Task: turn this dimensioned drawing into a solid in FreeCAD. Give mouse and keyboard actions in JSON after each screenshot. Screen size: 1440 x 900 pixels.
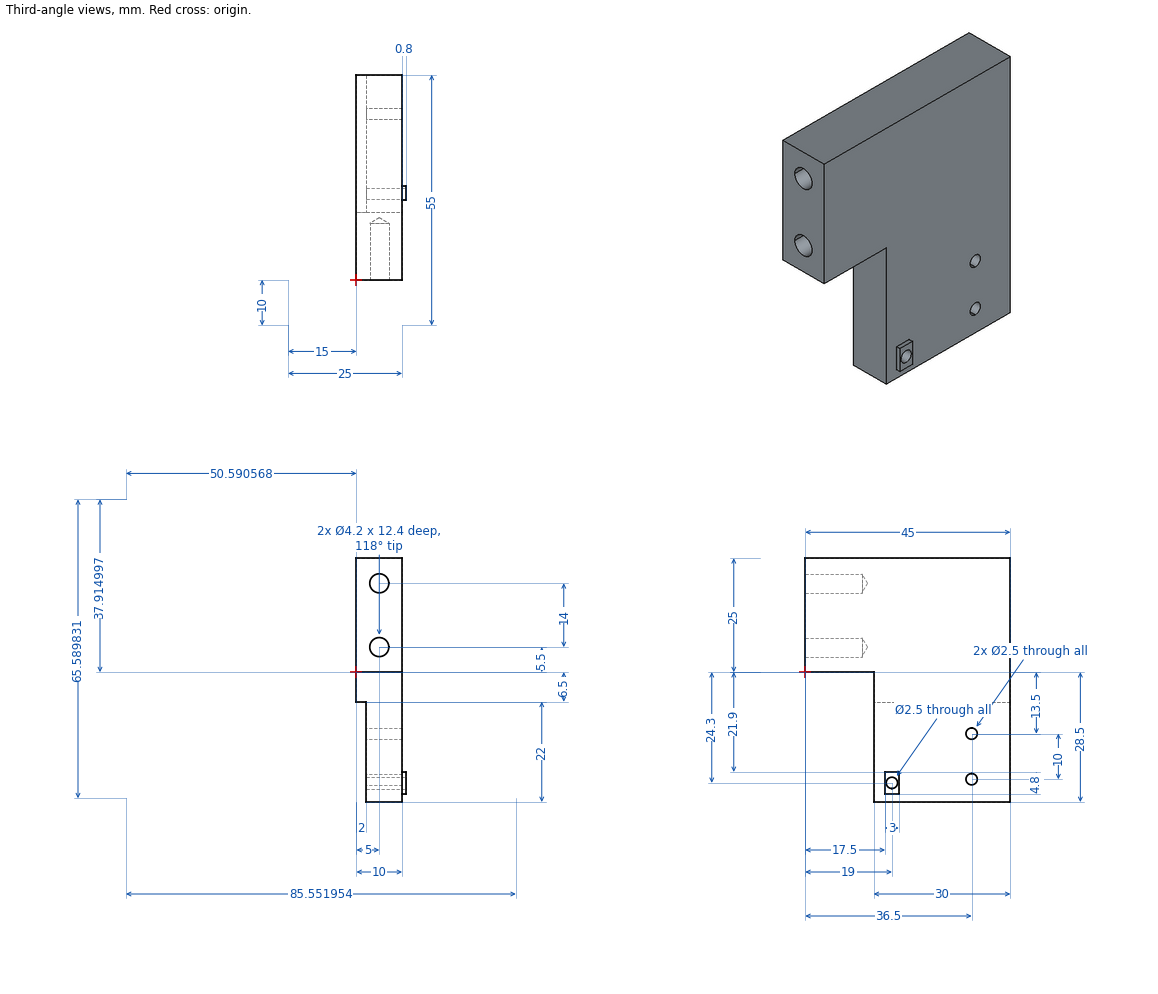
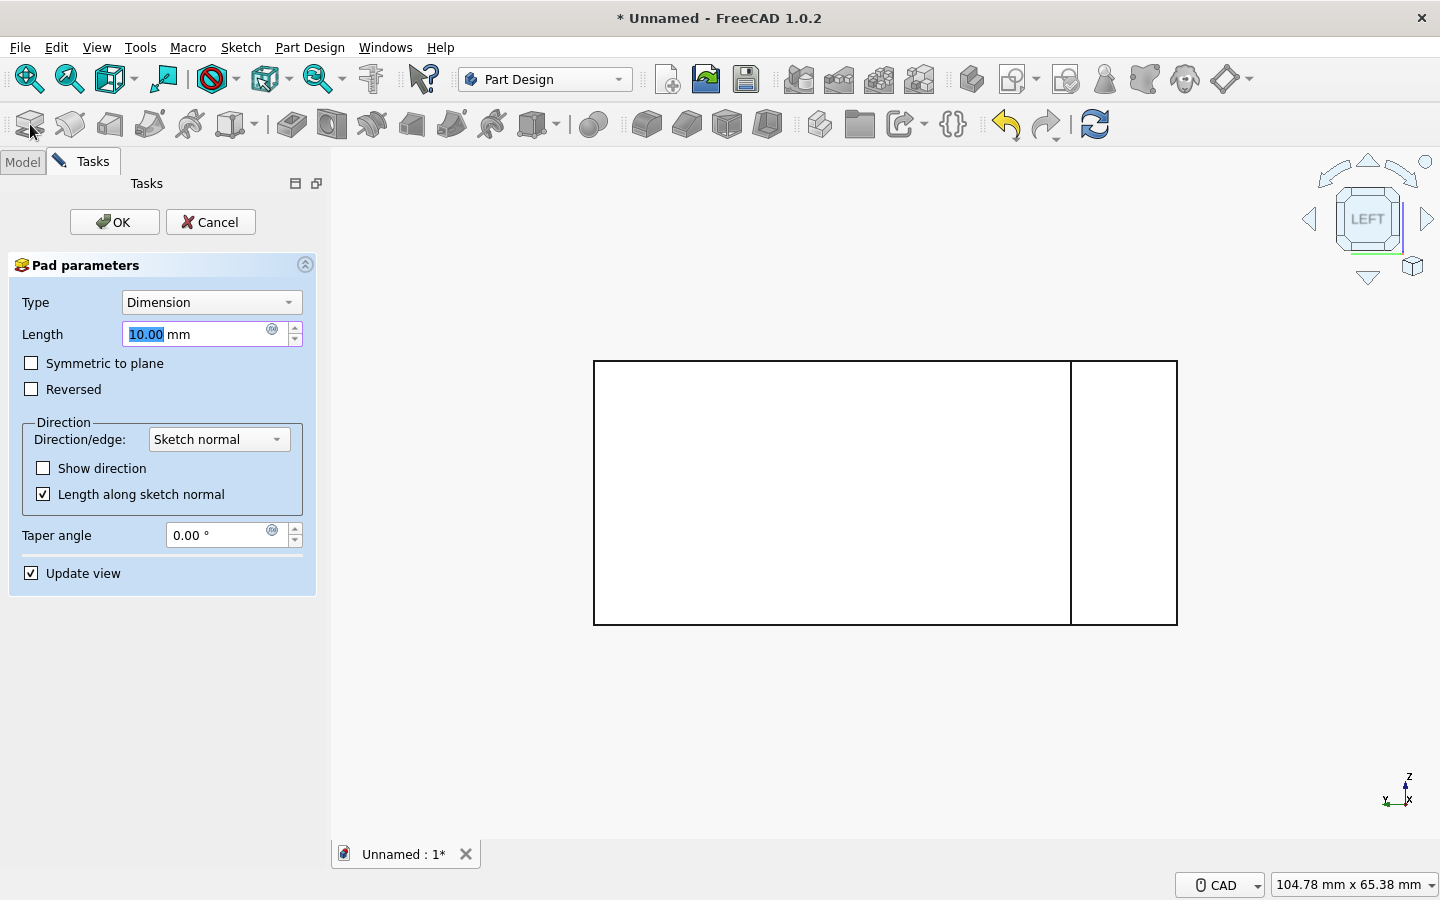
{"action": "type", "text": "10"}
{"action": "key", "text": "Tab"}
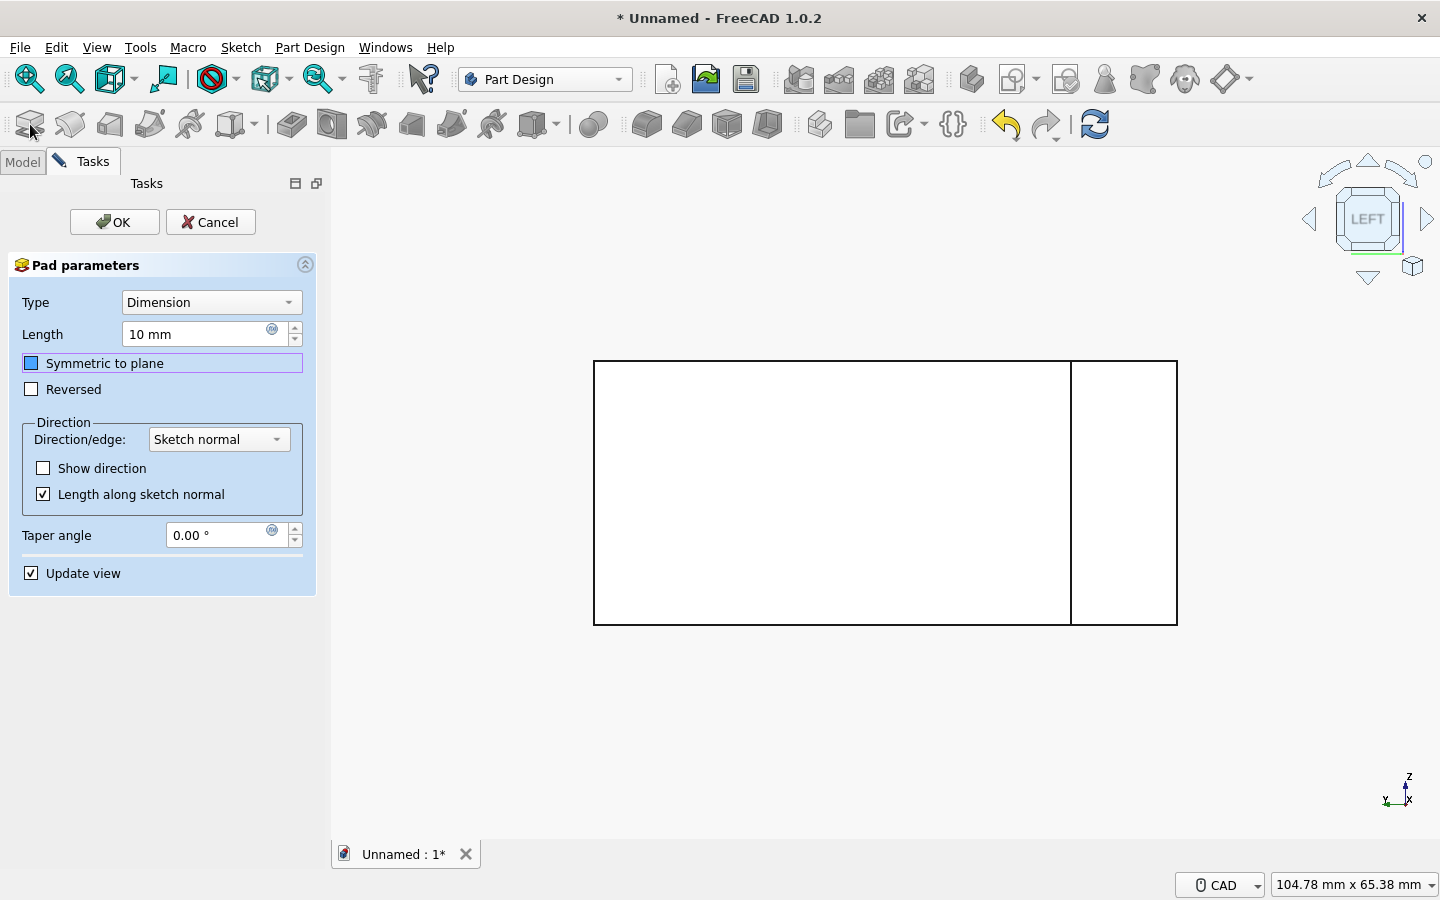
{"action": "left_click", "coordinate": [30, 389]}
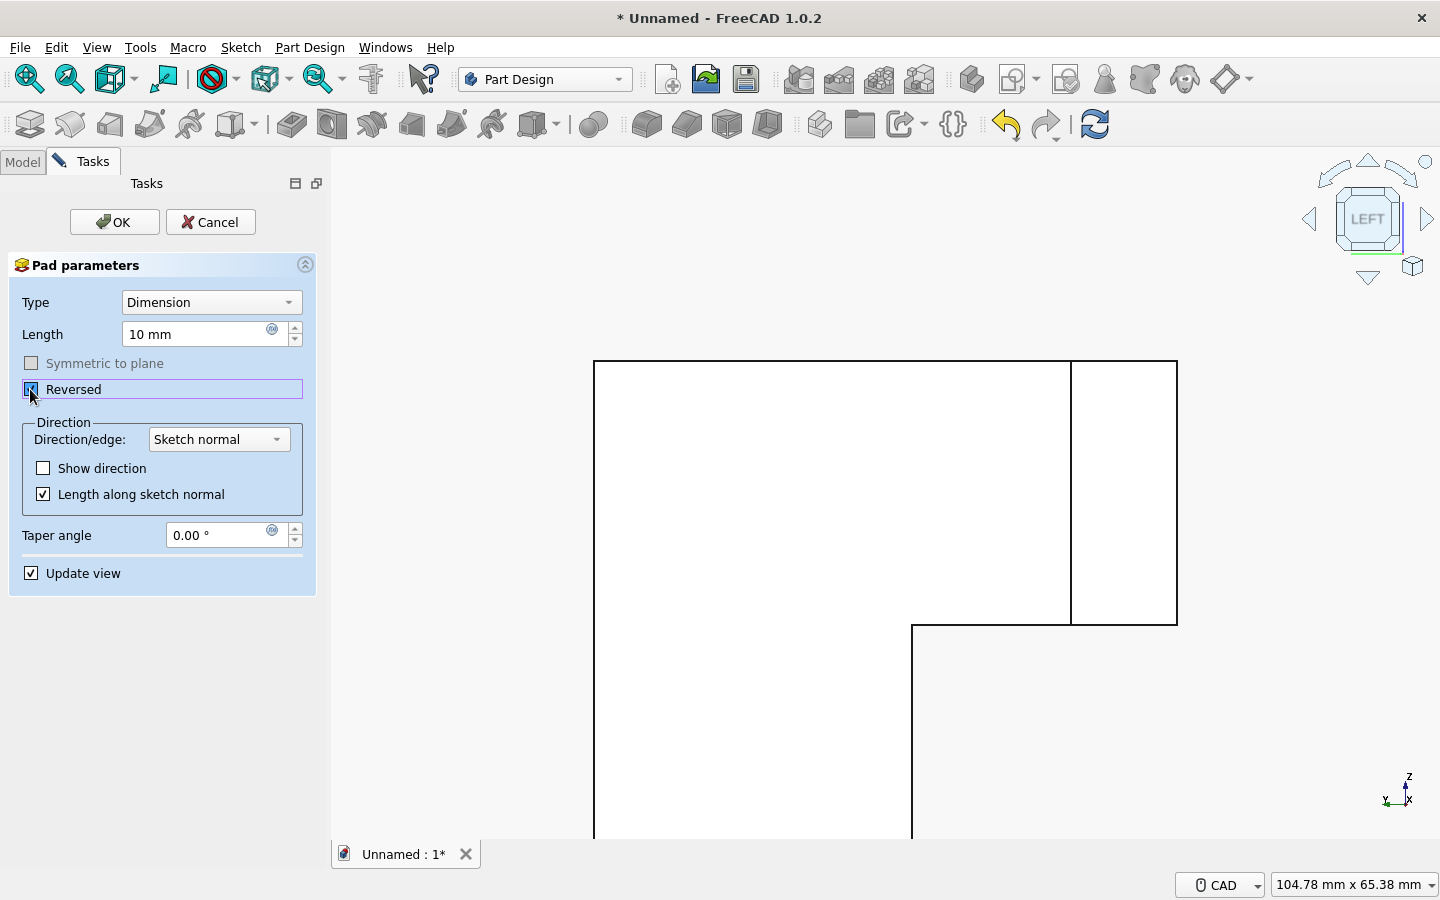
{"action": "left_click", "coordinate": [115, 222]}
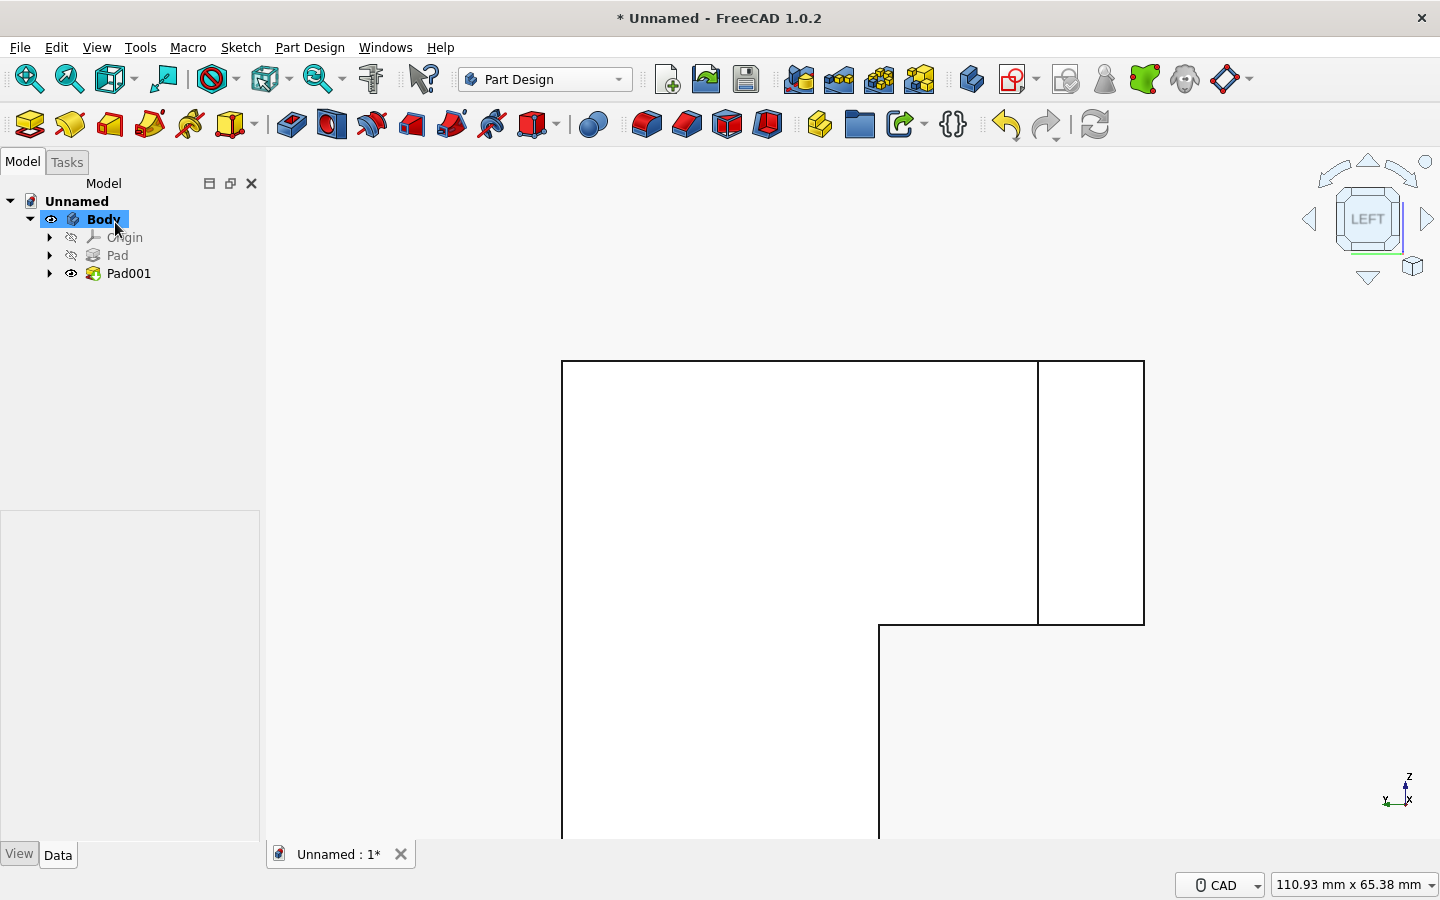
{"action": "key", "text": "v f"}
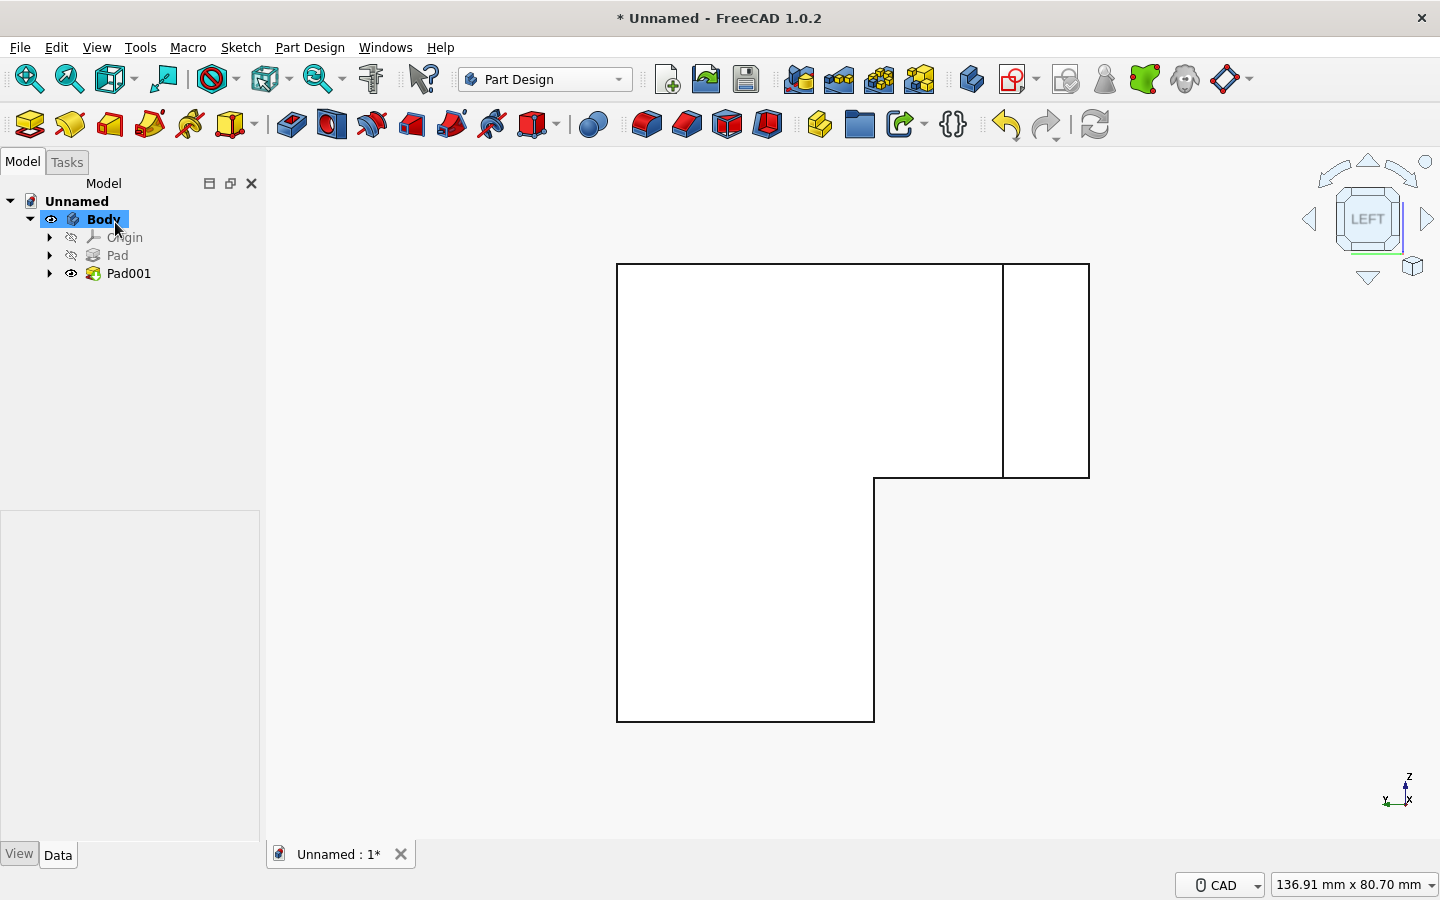
{"action": "key", "text": "4"}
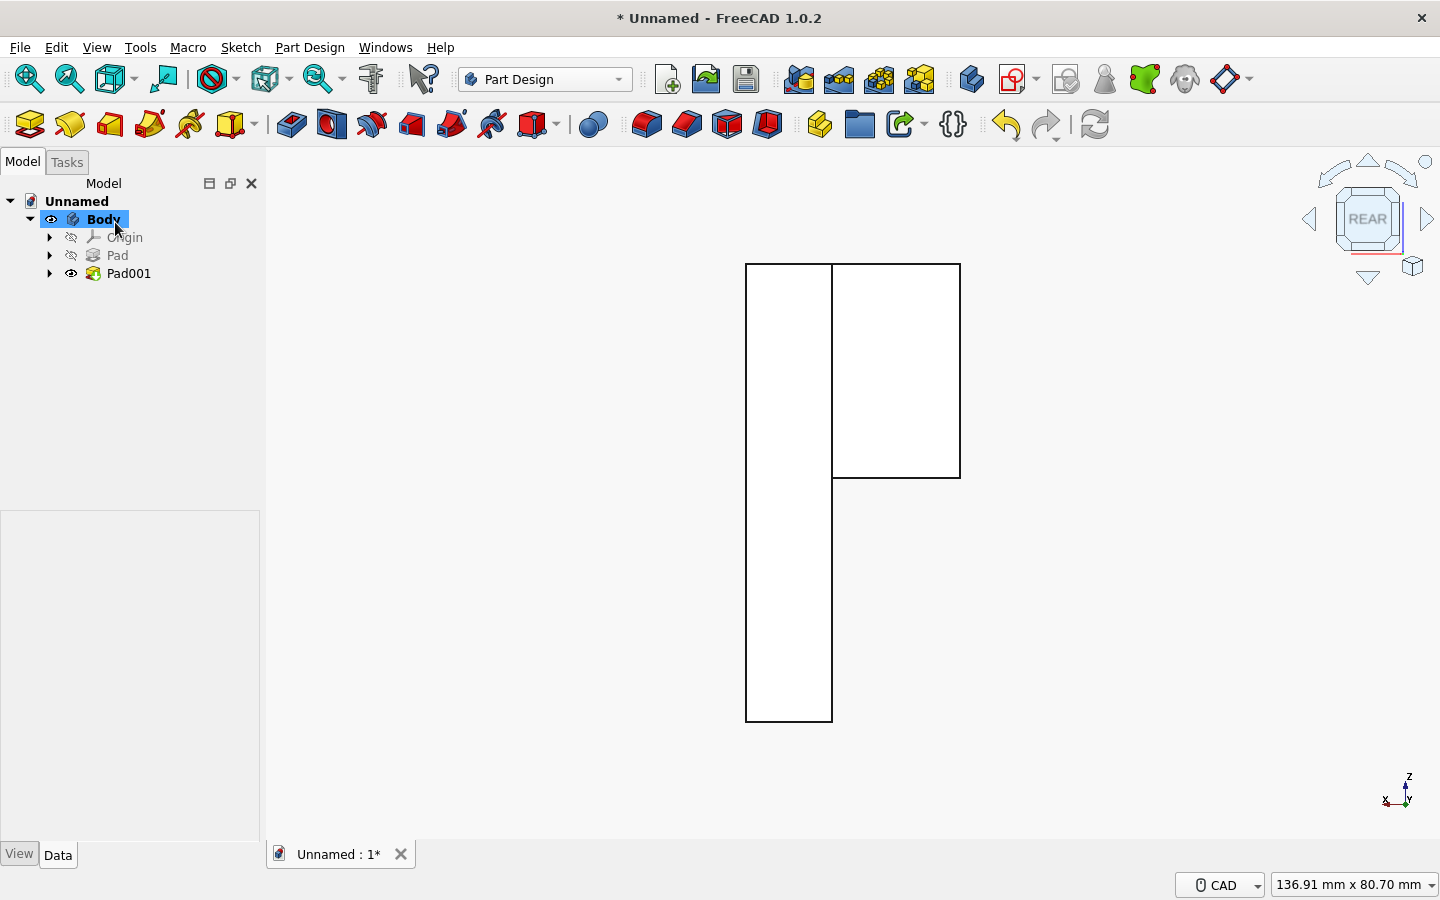
{"action": "left_click", "coordinate": [789, 361]}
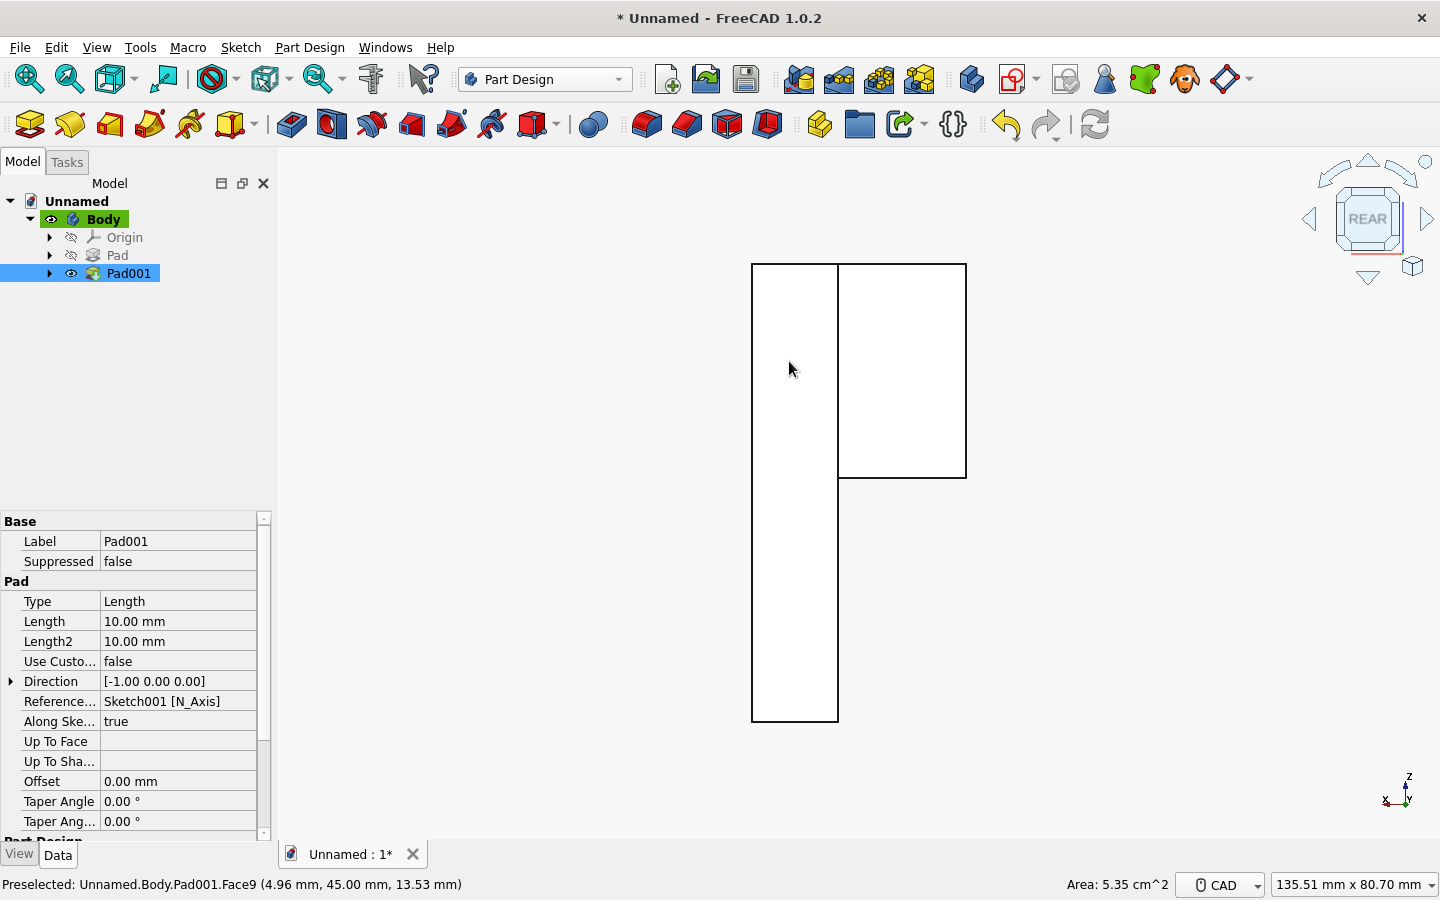
{"action": "left_click", "coordinate": [1012, 80]}